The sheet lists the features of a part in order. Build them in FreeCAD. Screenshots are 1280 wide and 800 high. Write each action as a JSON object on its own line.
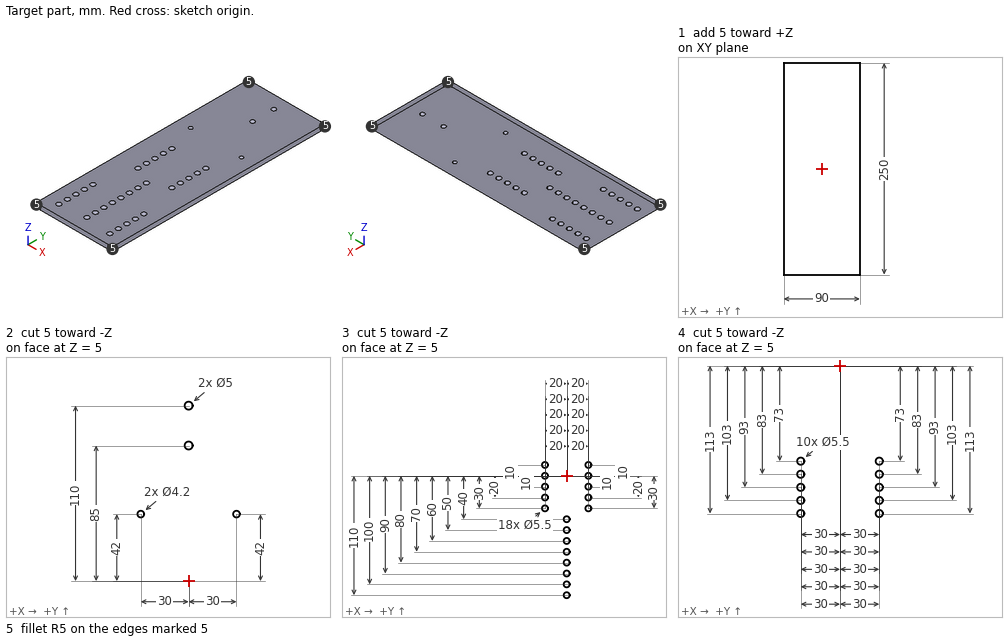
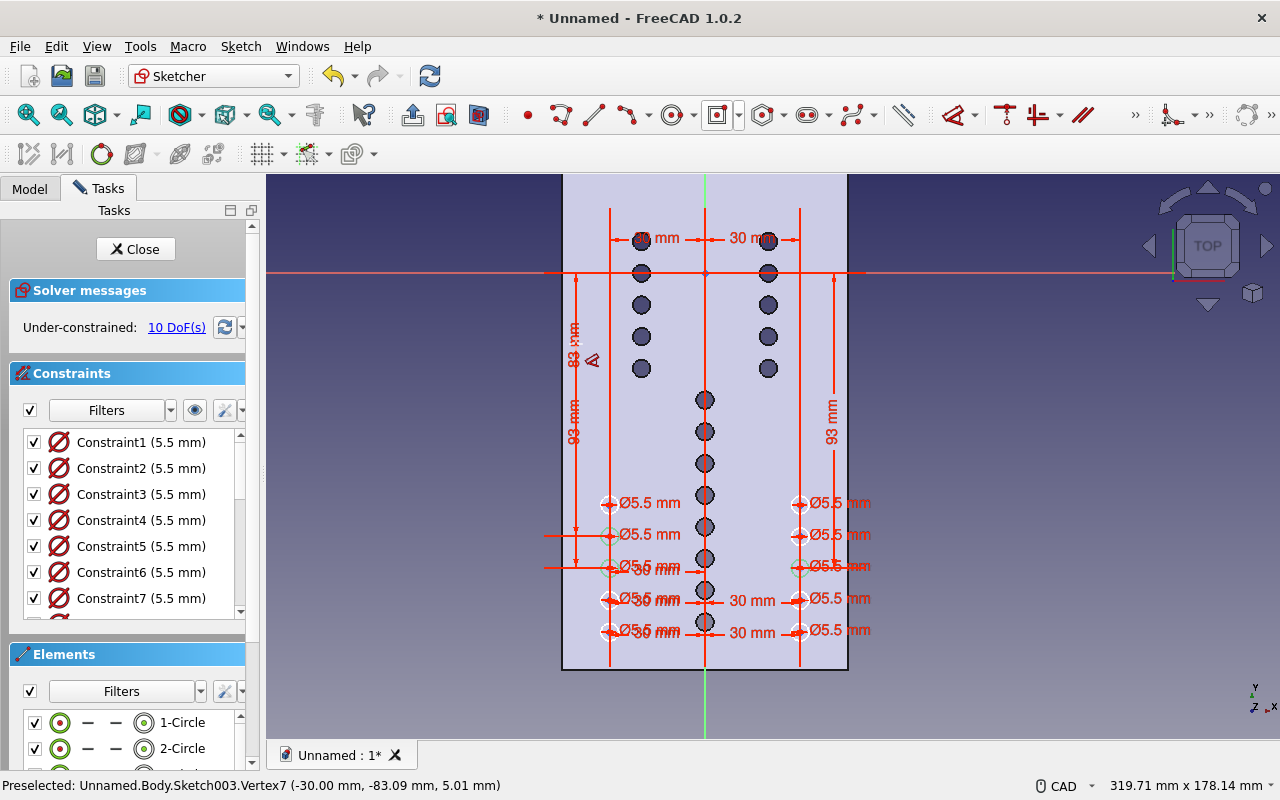
{"action": "left_click", "coordinate": [800, 537]}
{"action": "left_click", "coordinate": [753, 571]}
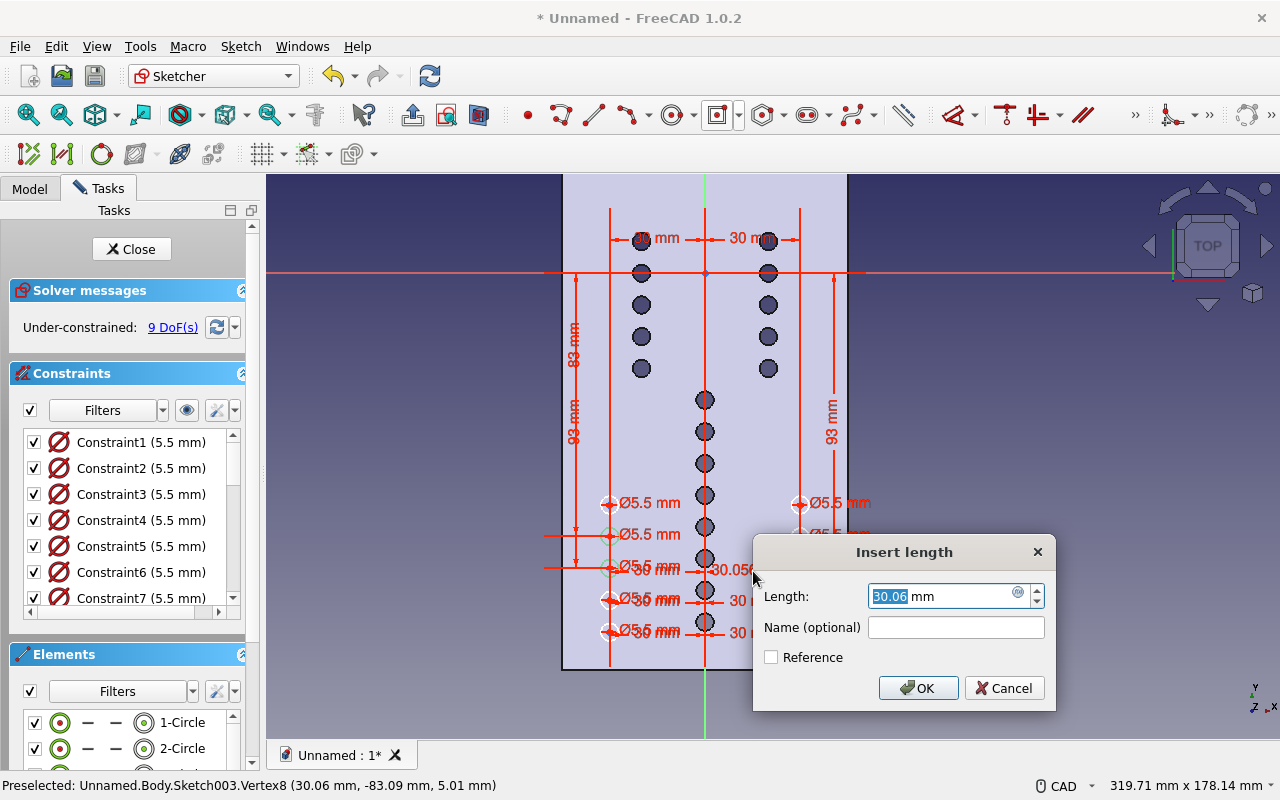
{"action": "type", "text": "30"}
{"action": "key", "text": "Return"}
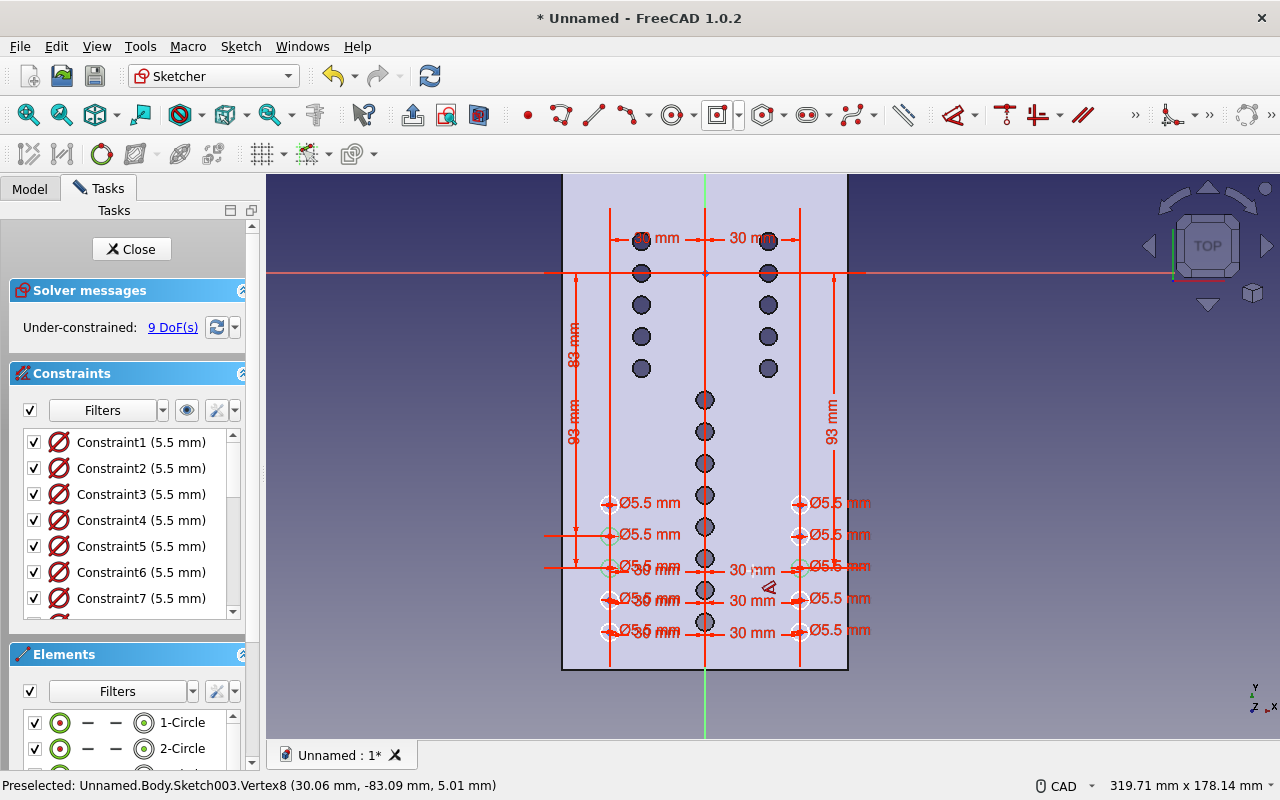
{"action": "left_click", "coordinate": [800, 537]}
{"action": "left_click", "coordinate": [834, 344]}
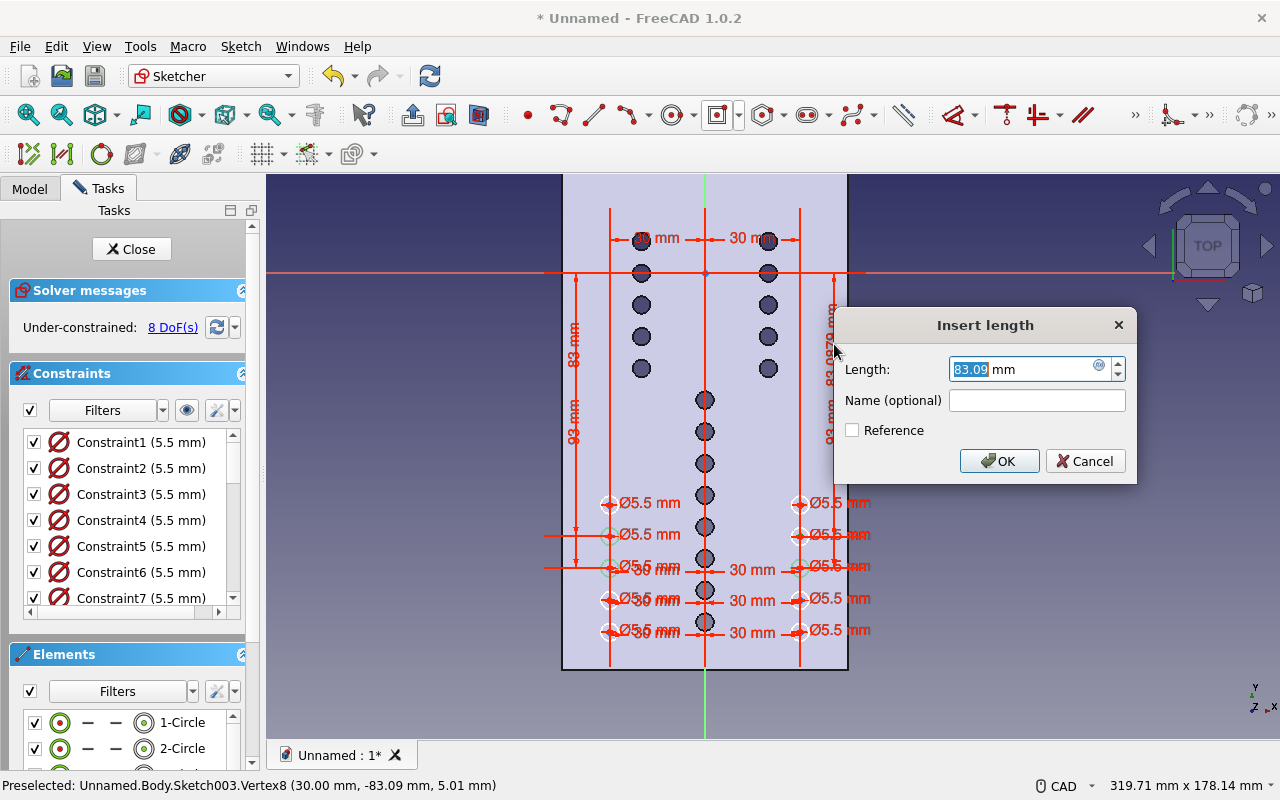
{"action": "type", "text": "83"}
{"action": "key", "text": "Return"}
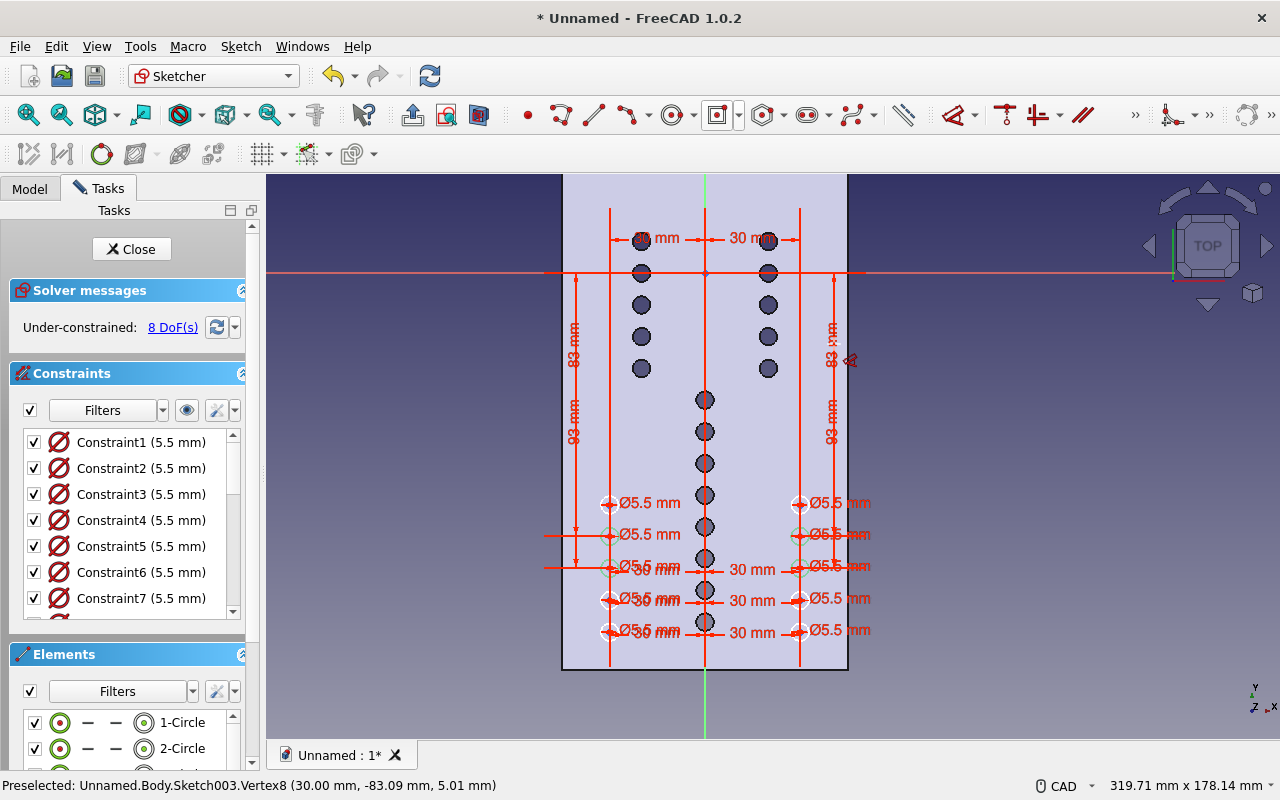
{"action": "left_click", "coordinate": [610, 505]}
{"action": "left_click", "coordinate": [657, 539]}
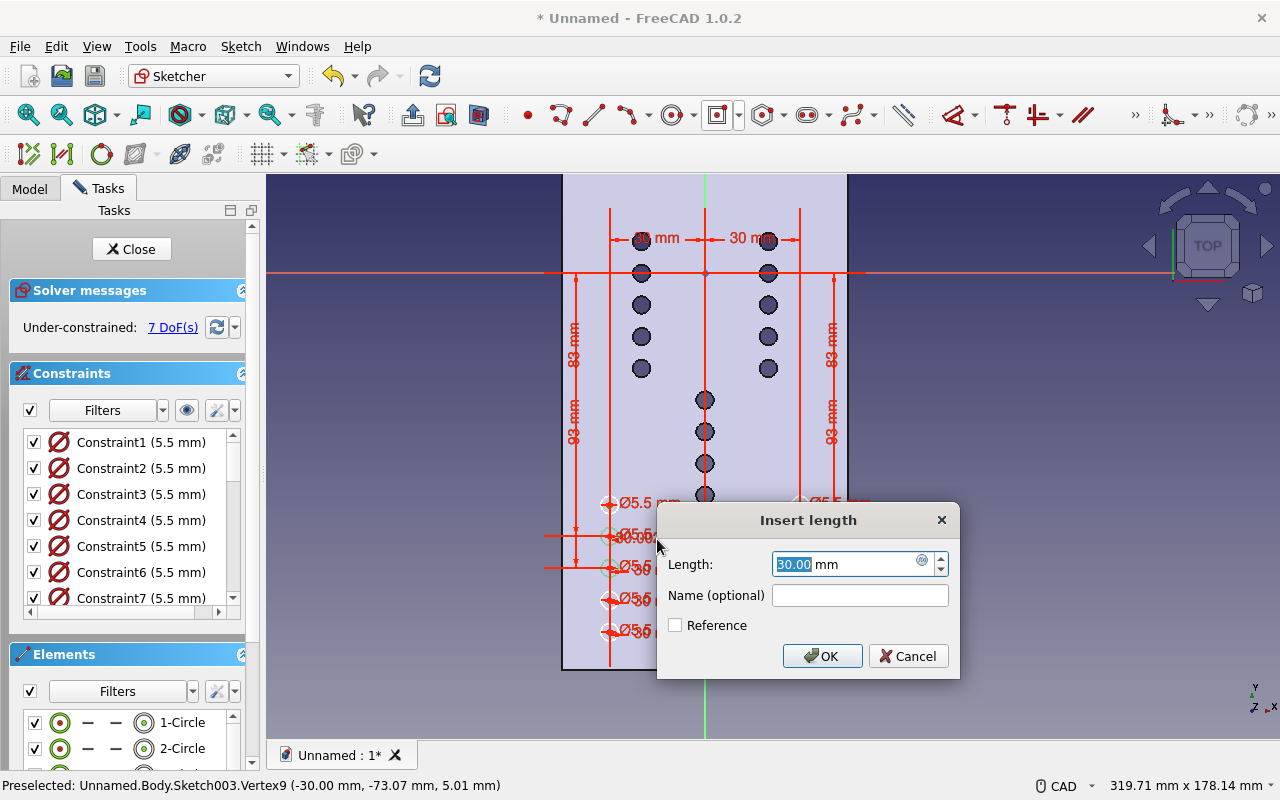
{"action": "type", "text": "30"}
{"action": "key", "text": "Return"}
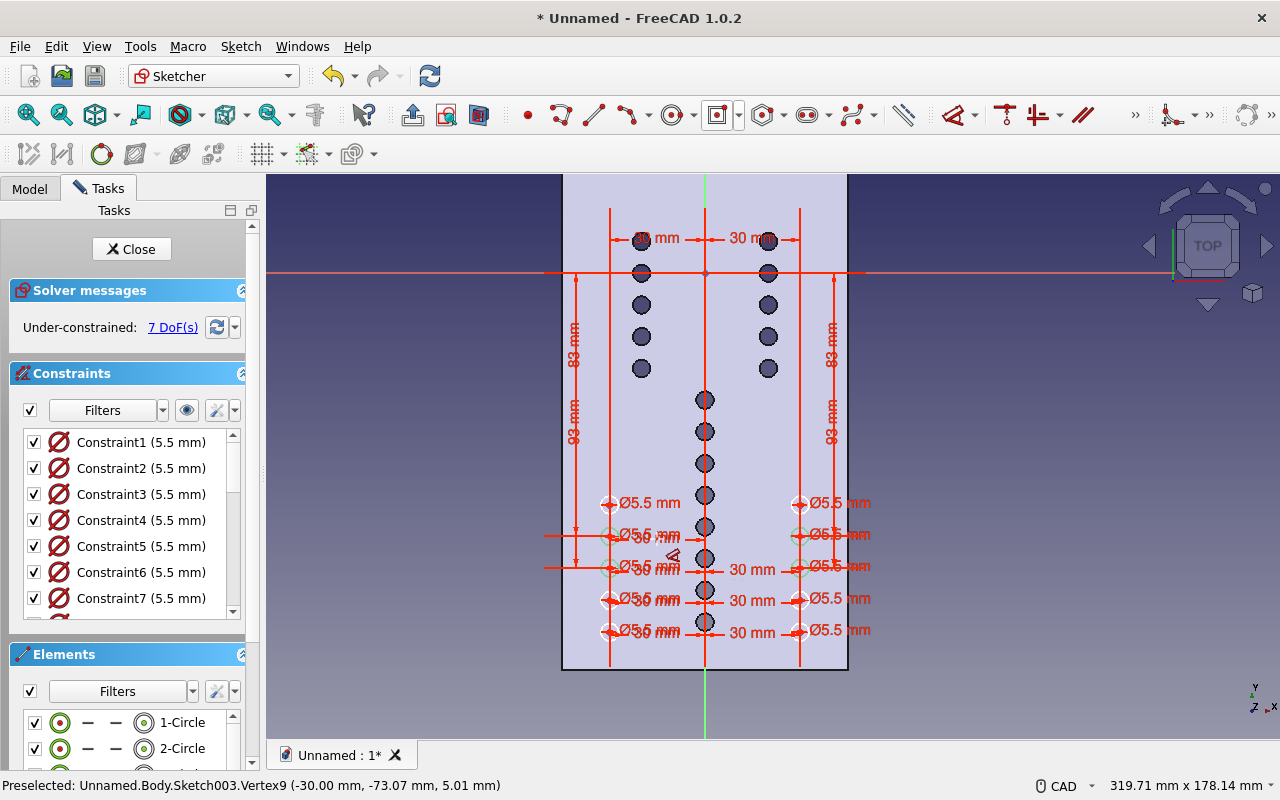
{"action": "left_click", "coordinate": [610, 505]}
{"action": "left_click", "coordinate": [576, 389]}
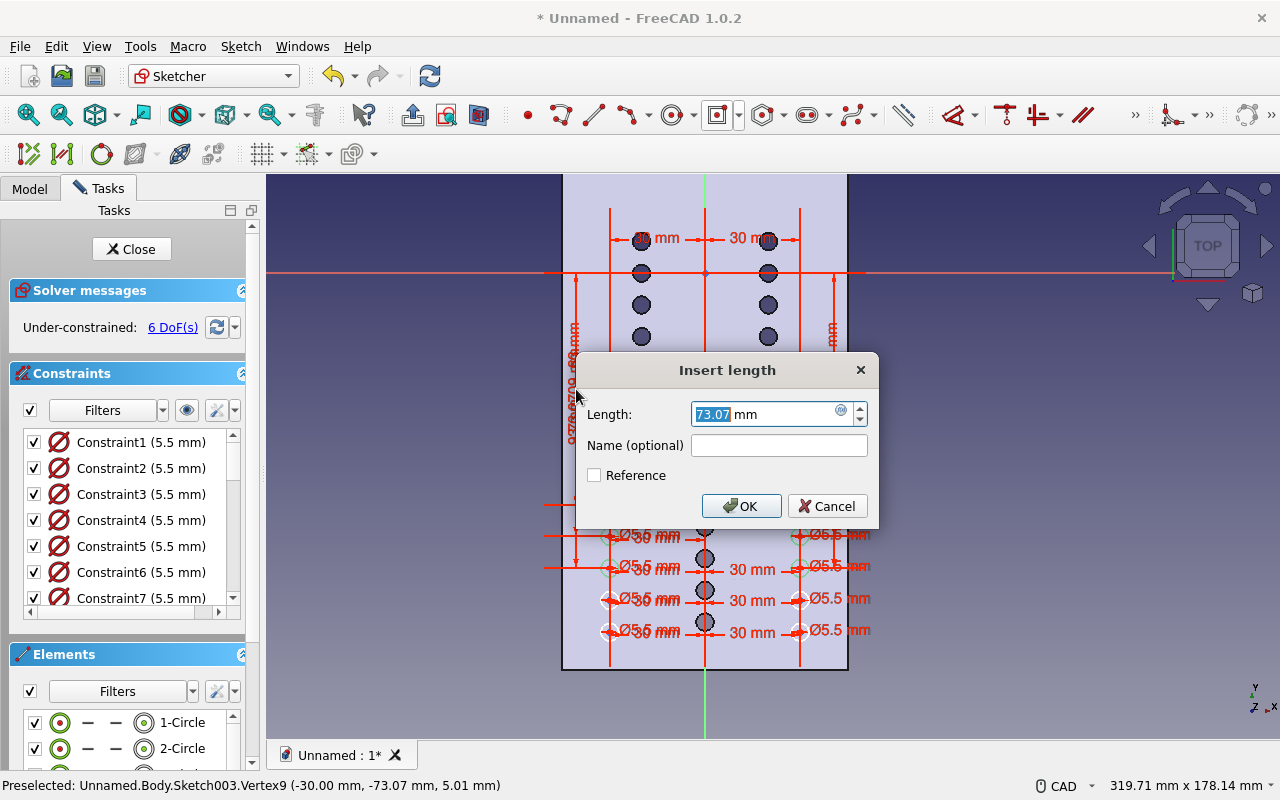
{"action": "type", "text": "73"}
{"action": "key", "text": "Return"}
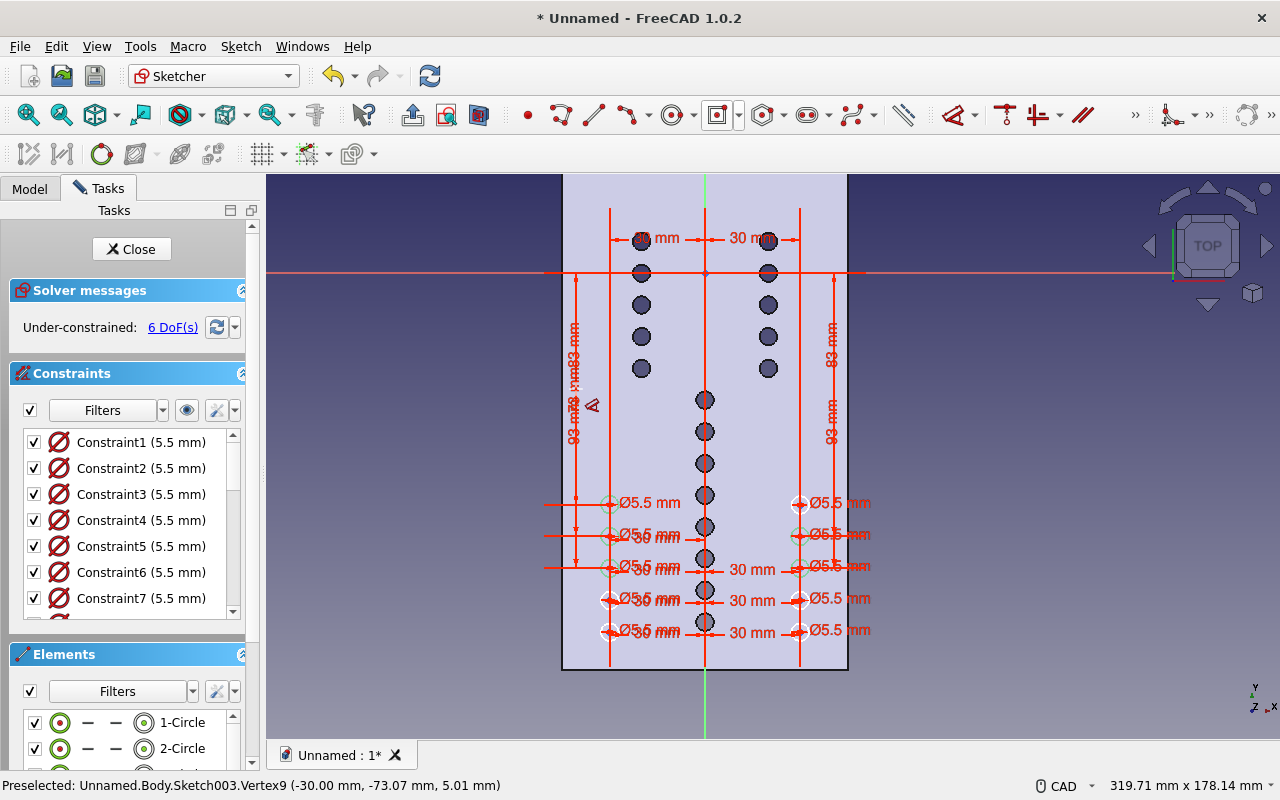
{"action": "left_click", "coordinate": [800, 505]}
{"action": "left_click", "coordinate": [753, 539]}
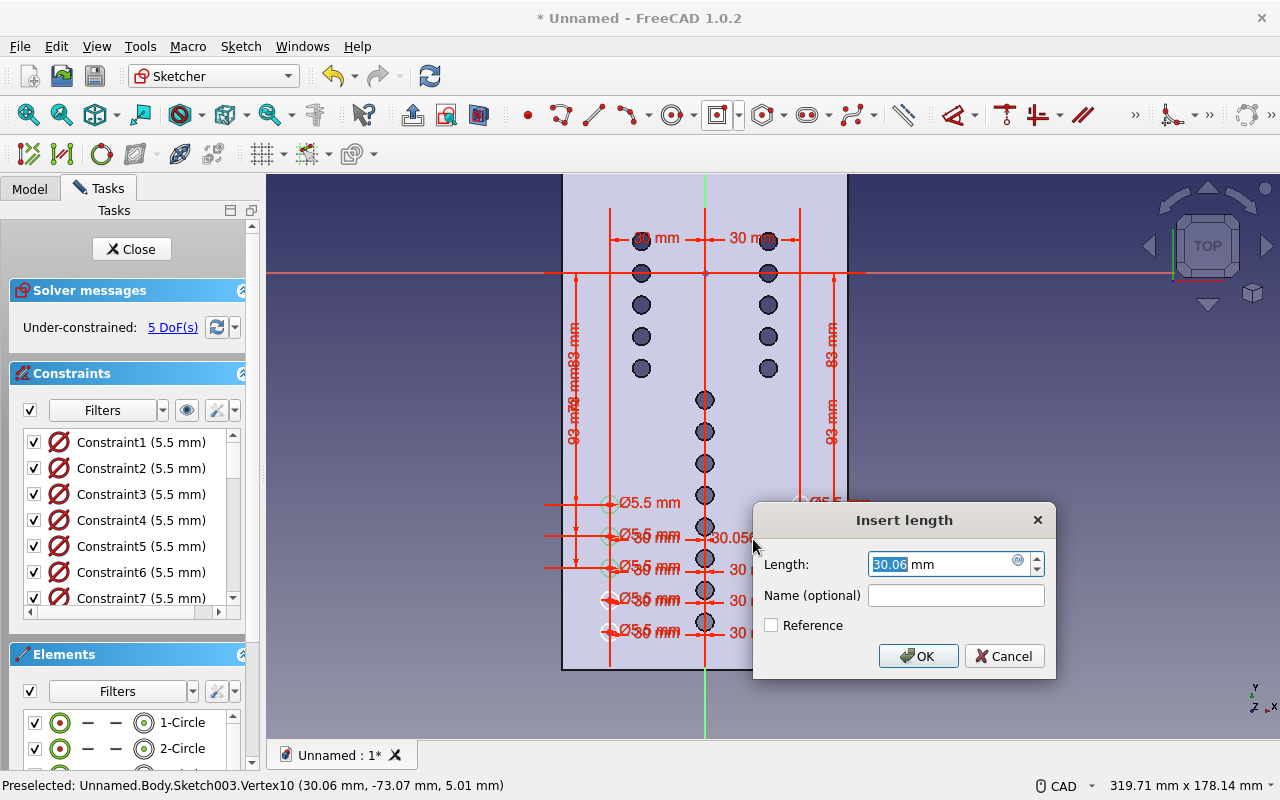
{"action": "type", "text": "30"}
{"action": "key", "text": "Return"}